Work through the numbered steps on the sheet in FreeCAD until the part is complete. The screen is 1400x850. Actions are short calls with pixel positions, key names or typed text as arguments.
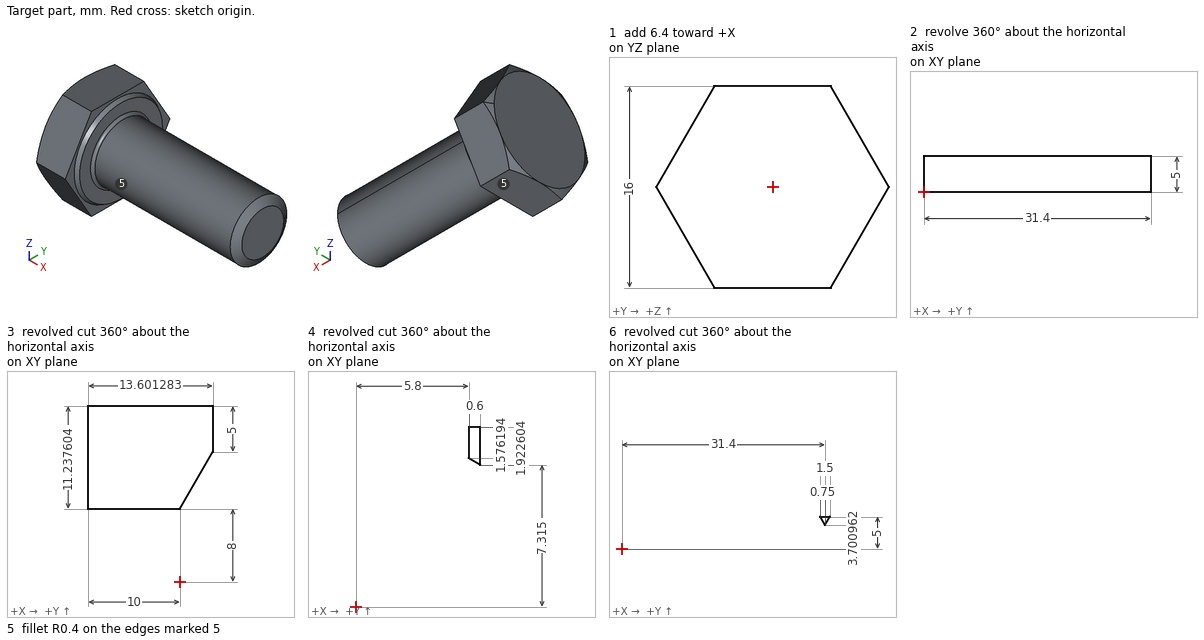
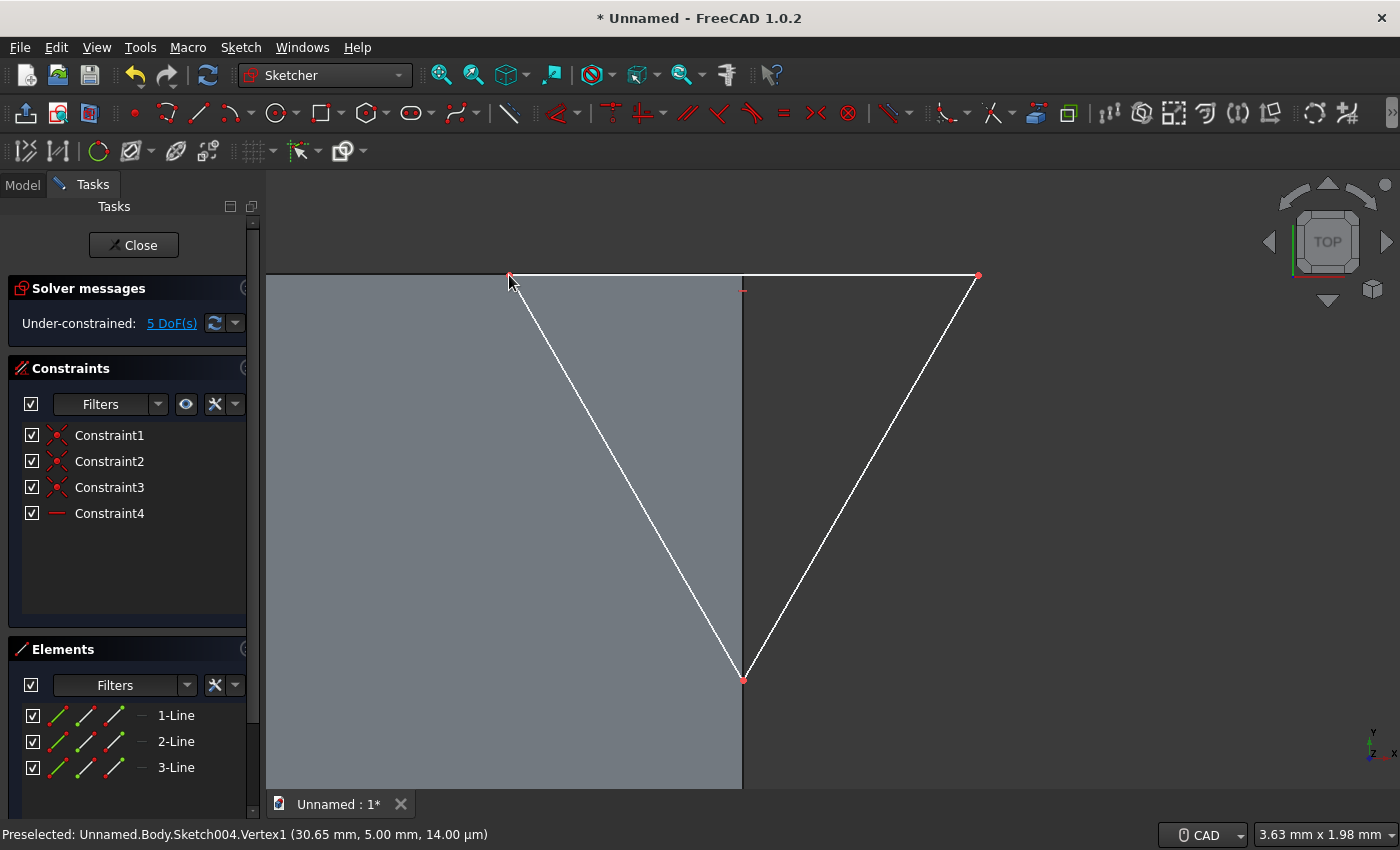
click(556, 114)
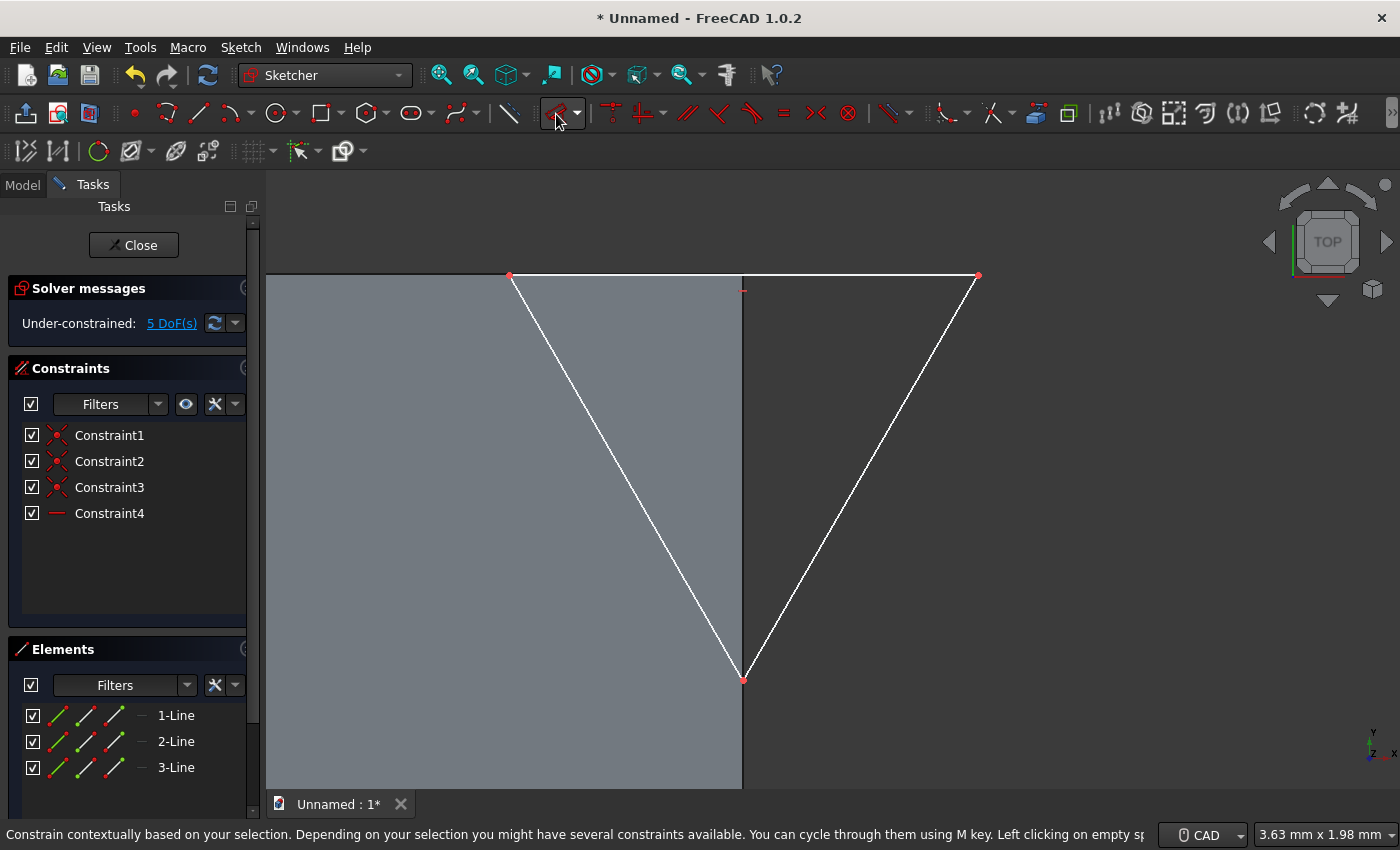
click(509, 275)
click(543, 518)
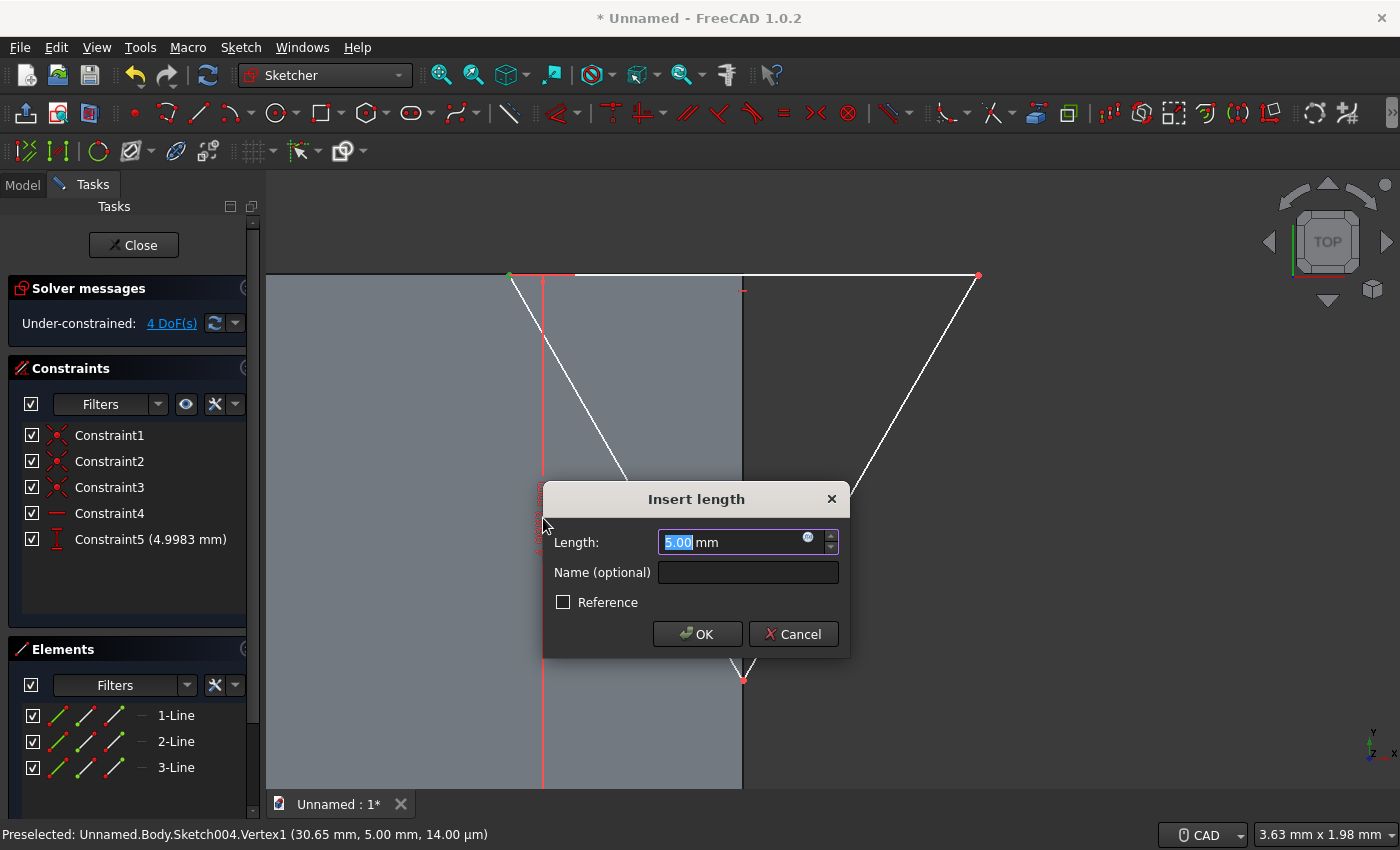
text(5)
key(Return)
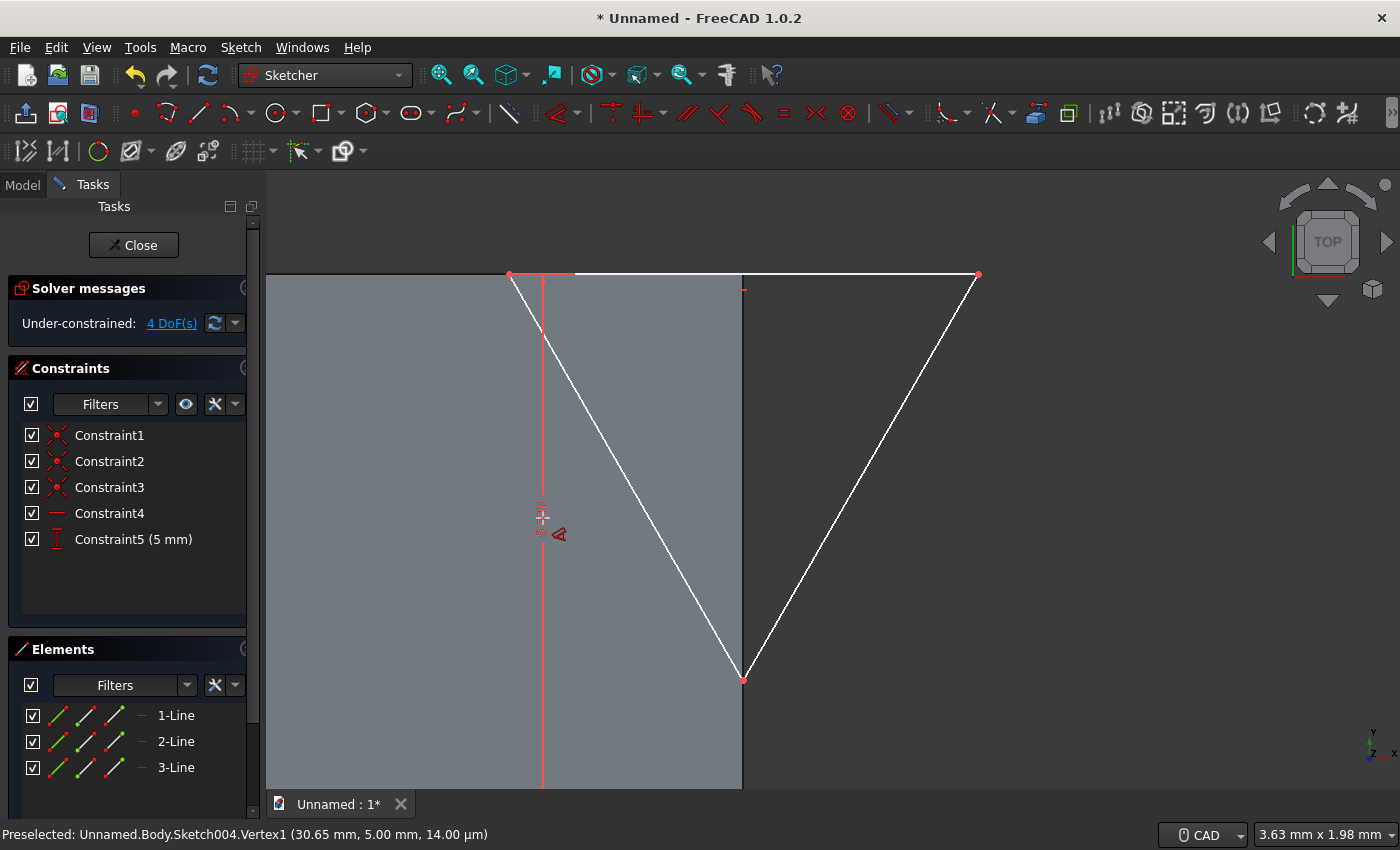
click(837, 274)
click(744, 240)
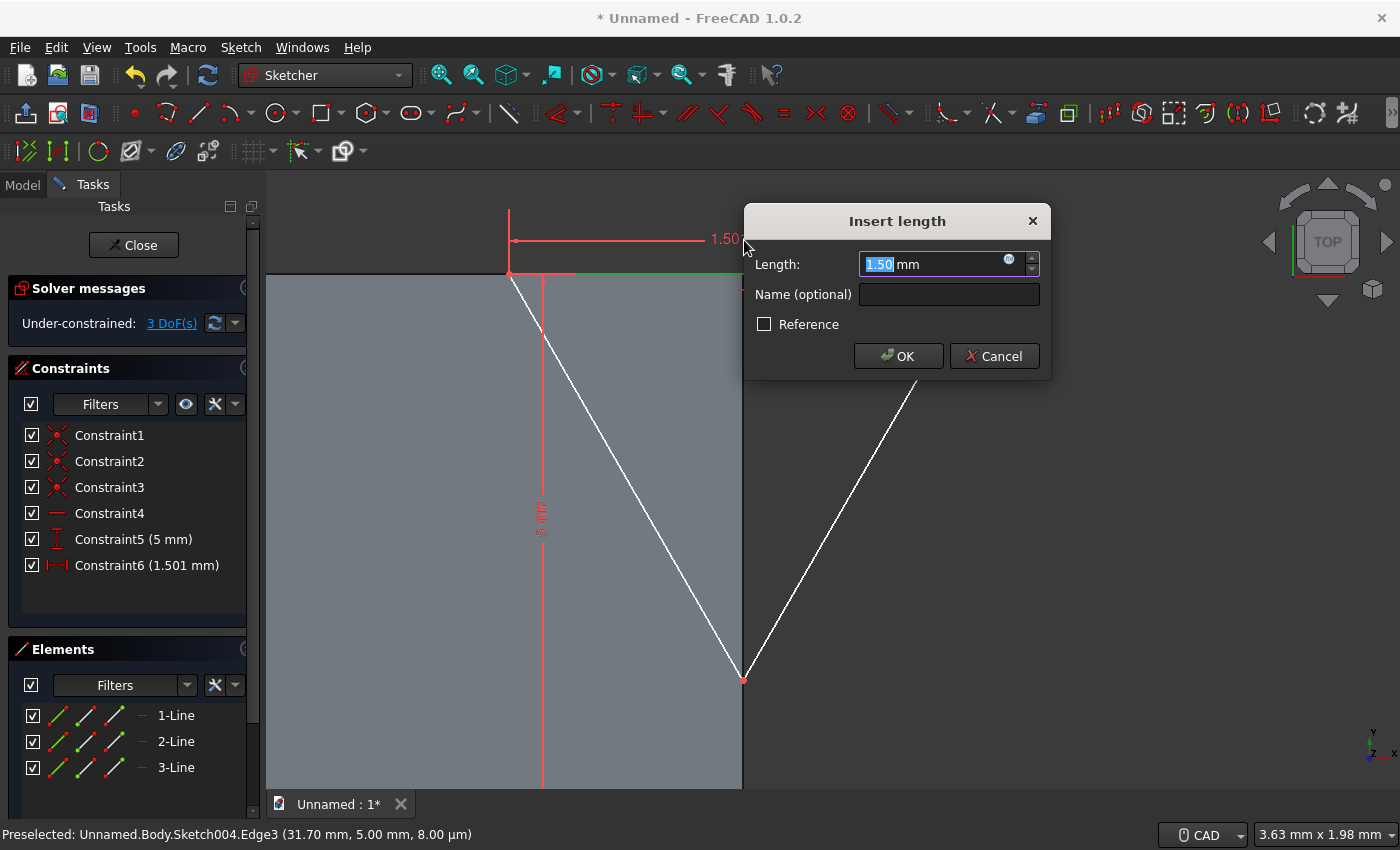
text(1.5)
key(Return)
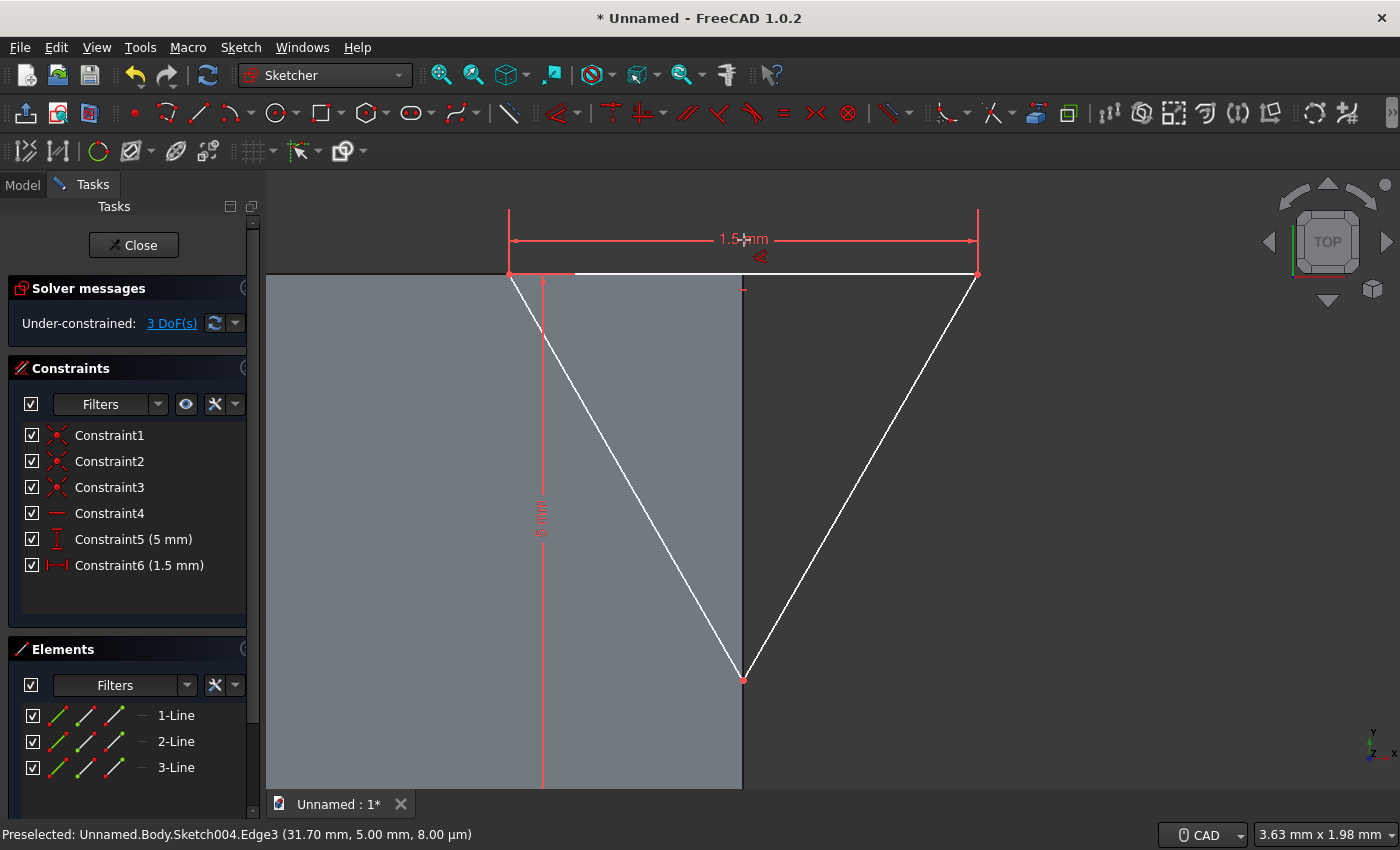
click(743, 681)
click(518, 647)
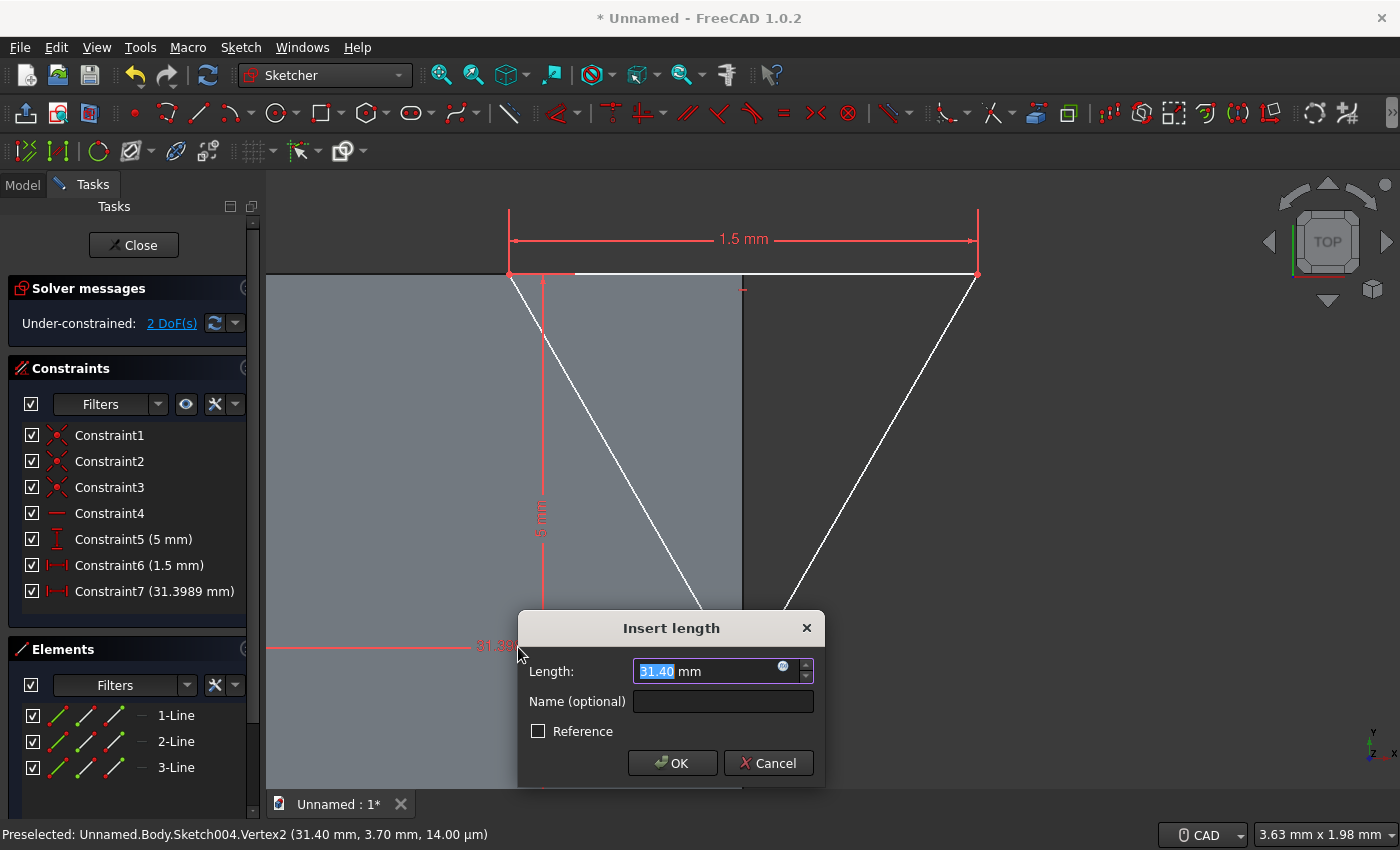
text(31.4)
key(Return)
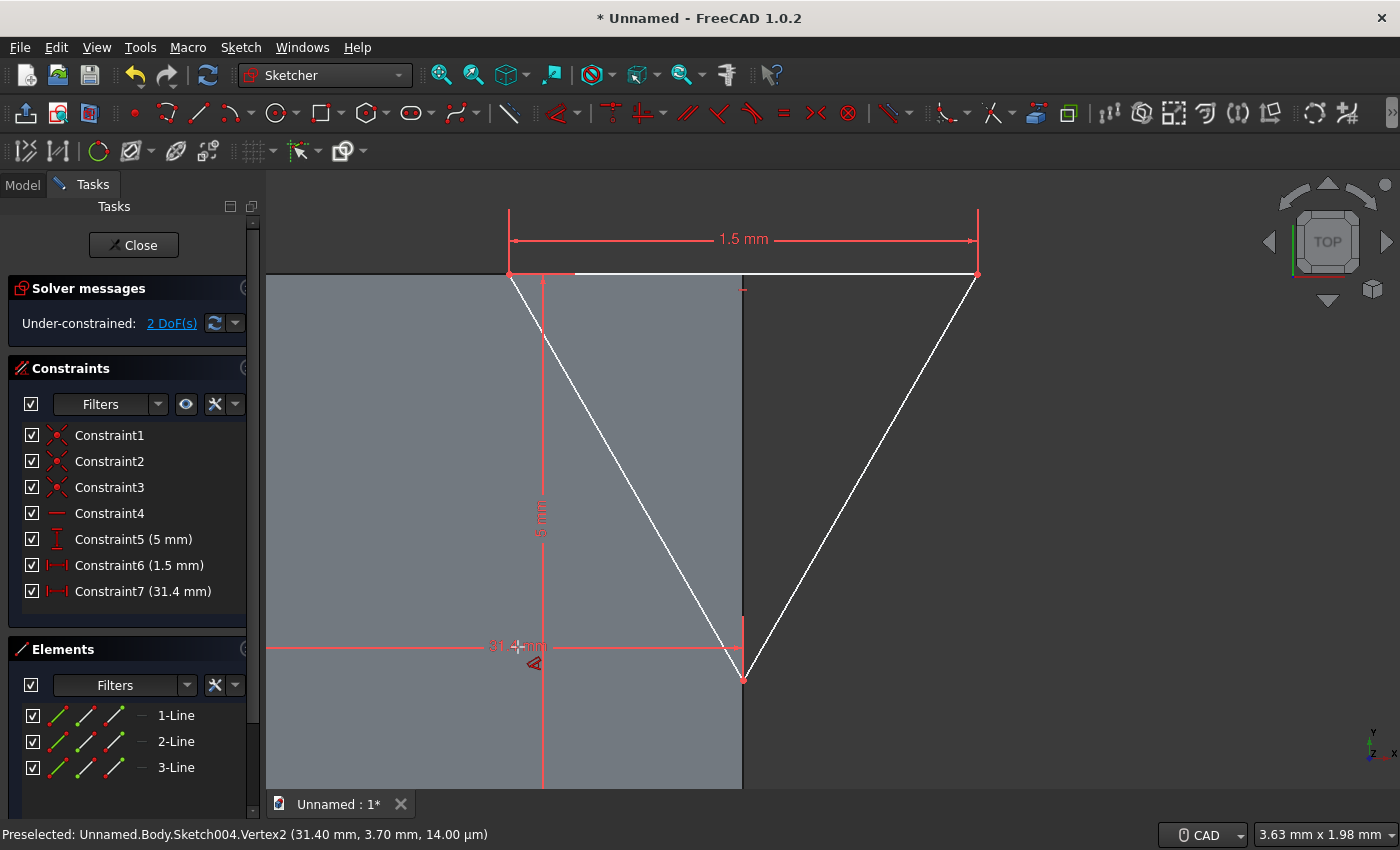
click(579, 396)
click(626, 715)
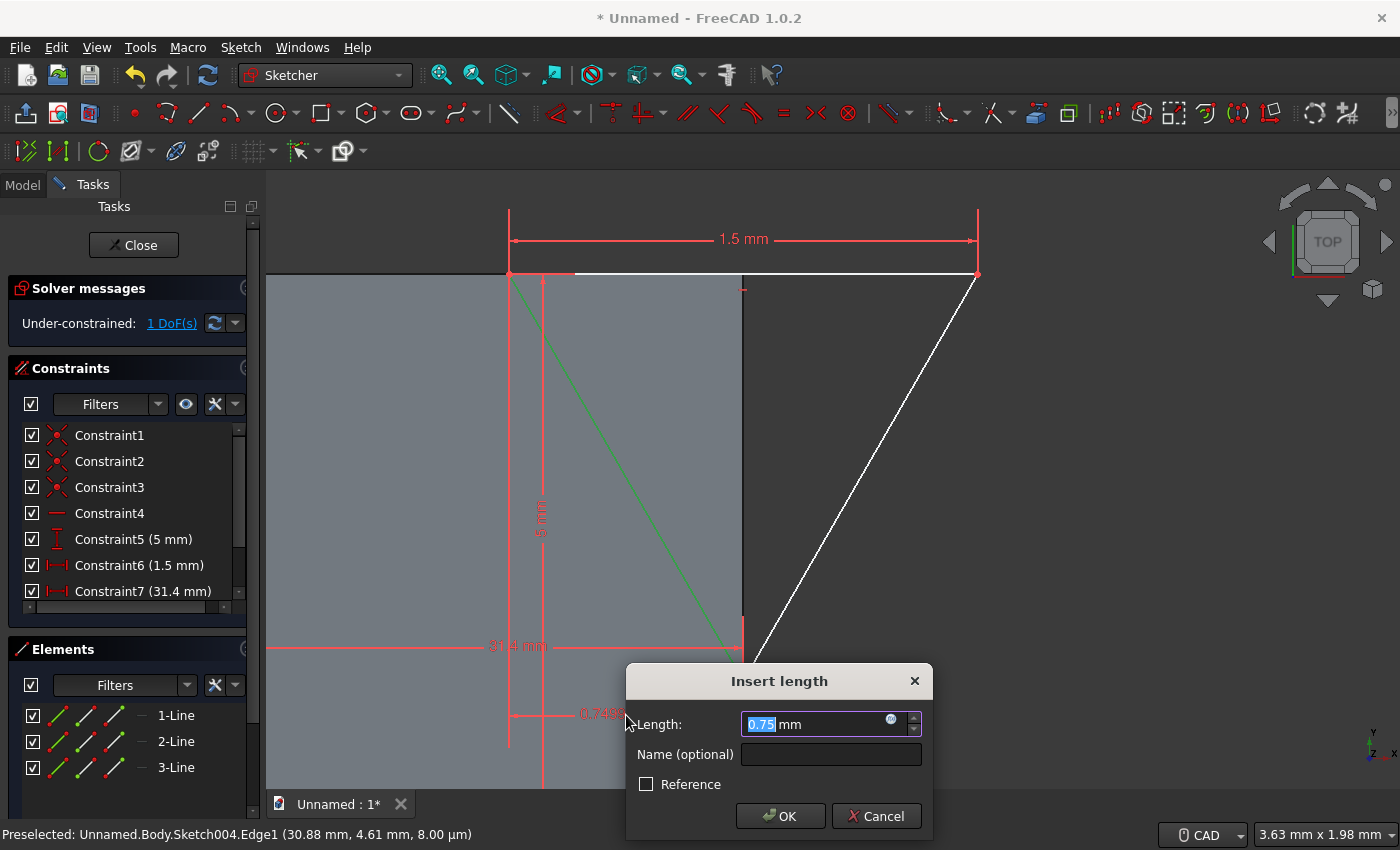
text(0.75)
key(Return)